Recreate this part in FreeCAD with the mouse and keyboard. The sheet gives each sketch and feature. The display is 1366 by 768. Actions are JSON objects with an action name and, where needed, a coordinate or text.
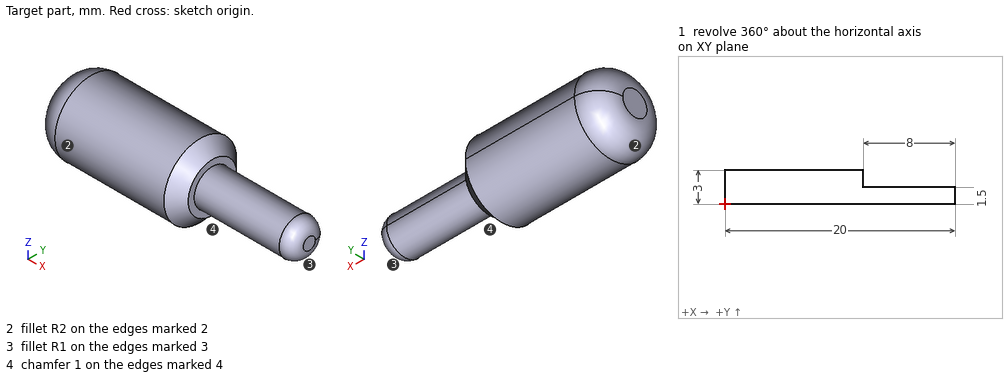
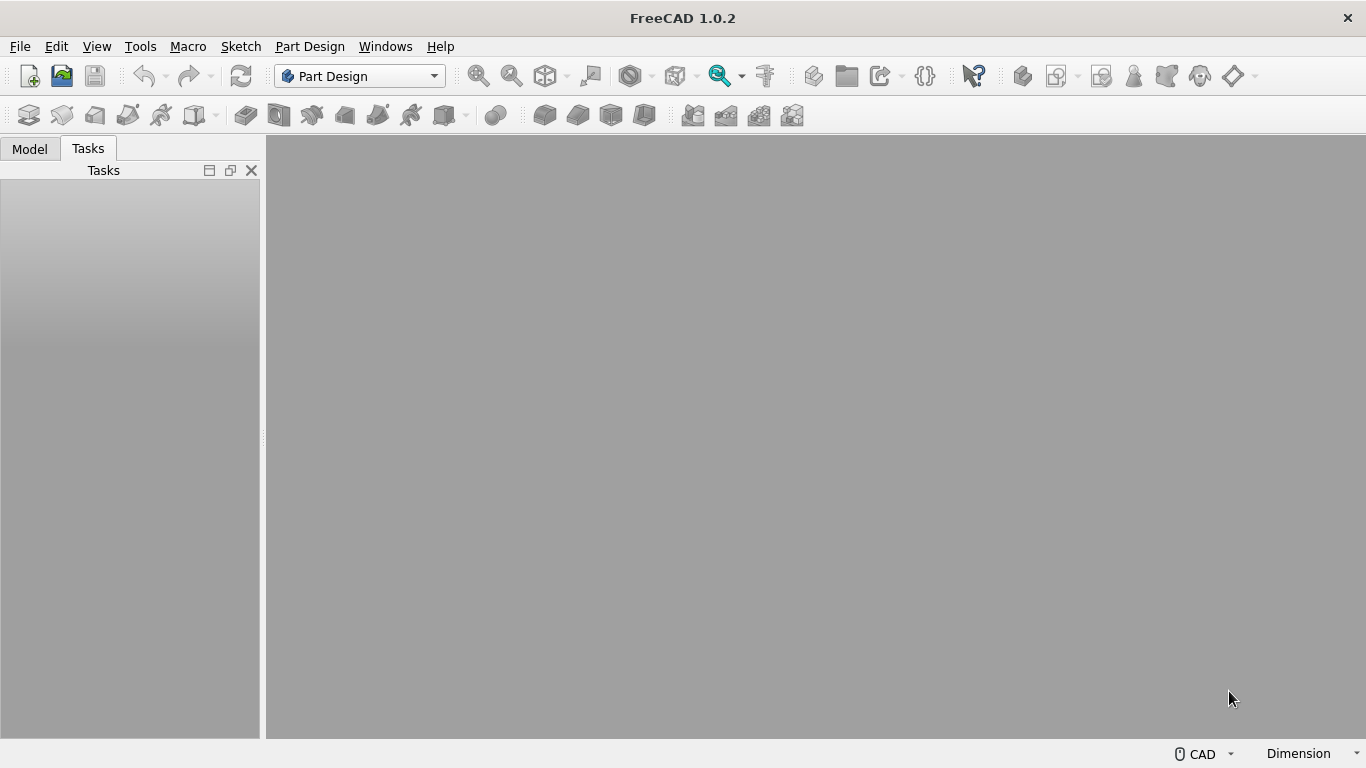
{"action": "key", "text": "ctrl+n"}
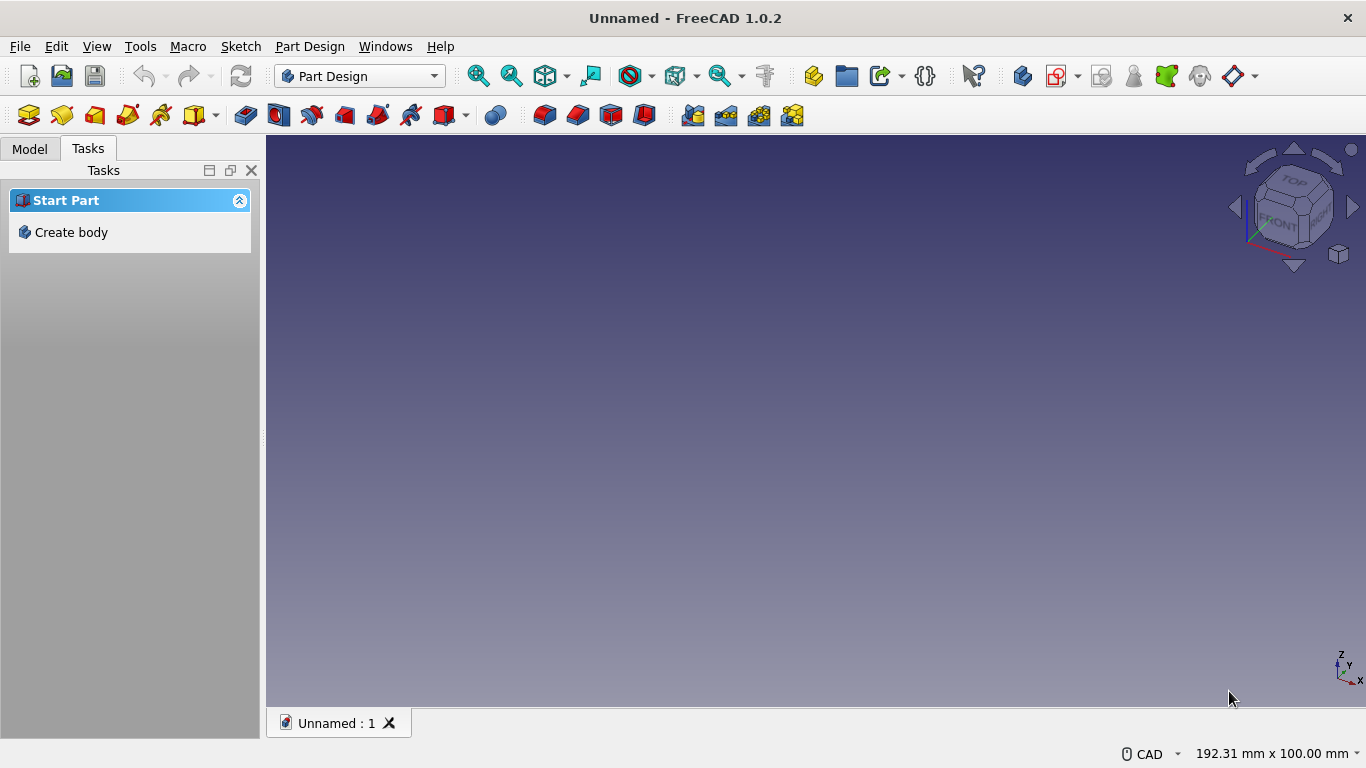
{"action": "left_click", "coordinate": [1056, 76]}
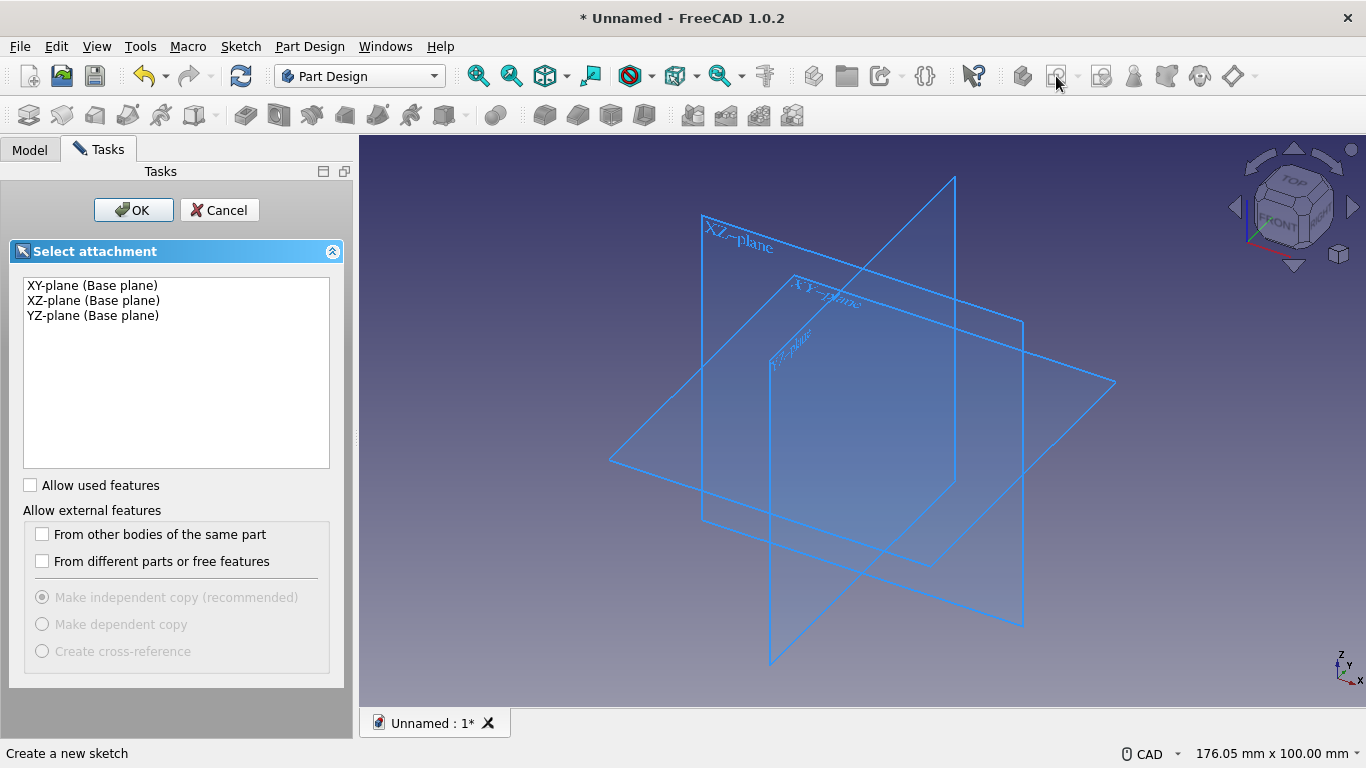
{"action": "left_click", "coordinate": [84, 286]}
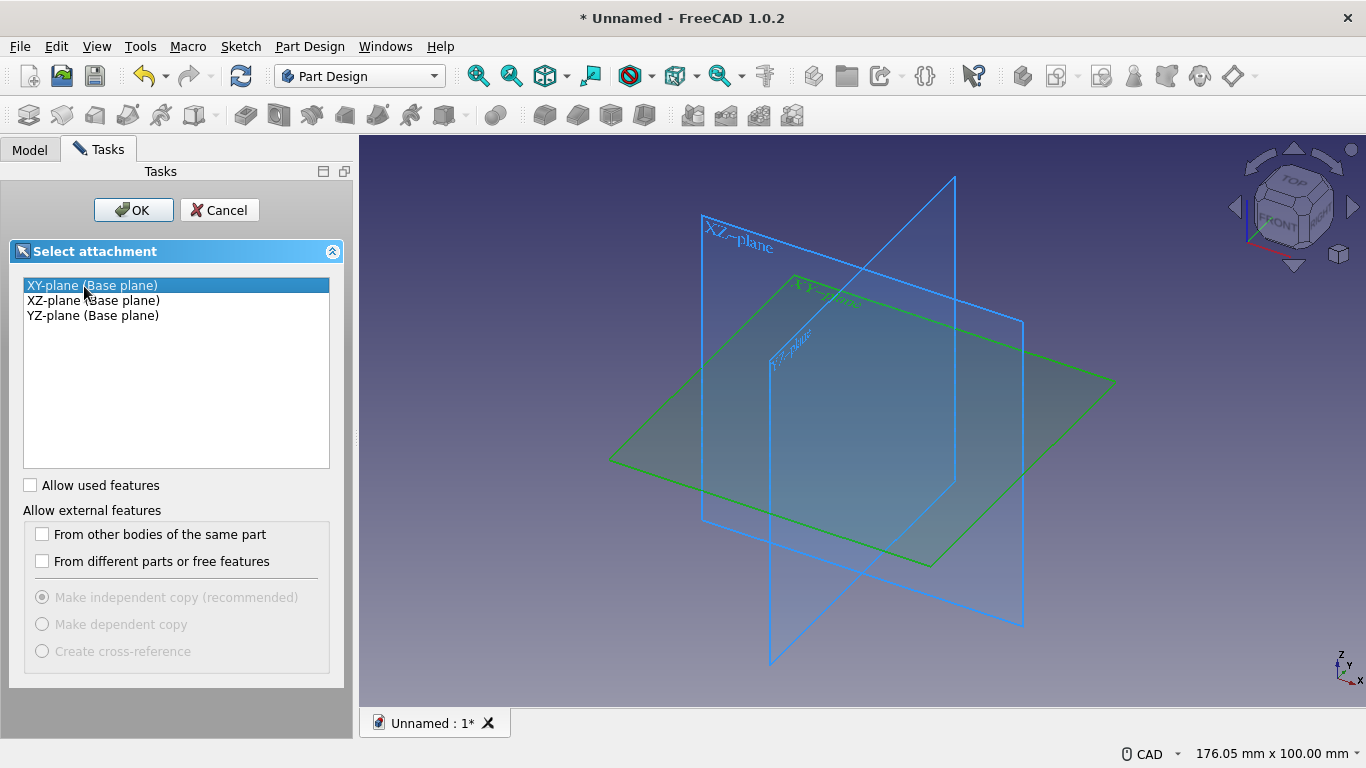
{"action": "left_click", "coordinate": [134, 210]}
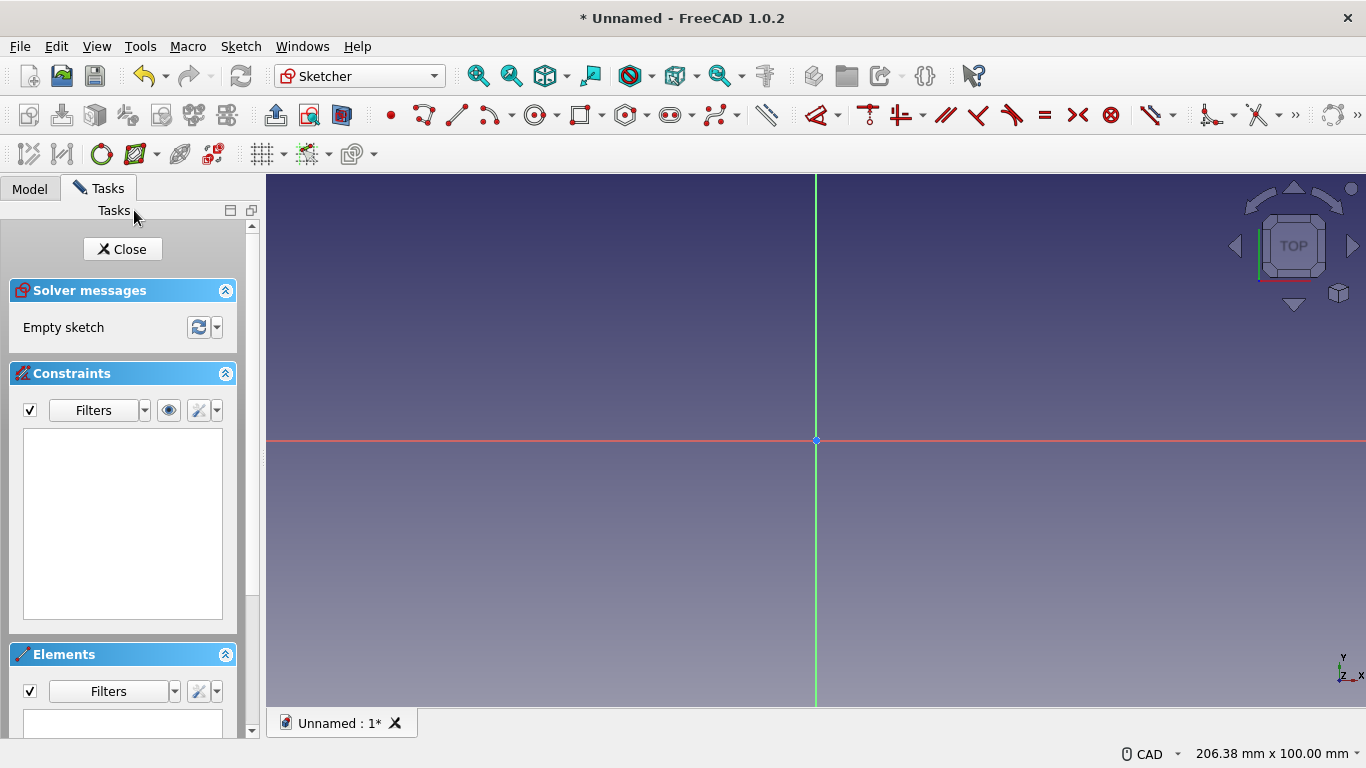
{"action": "scroll", "coordinate": [893, 431], "scroll_direction": "up", "scroll_amount": 9}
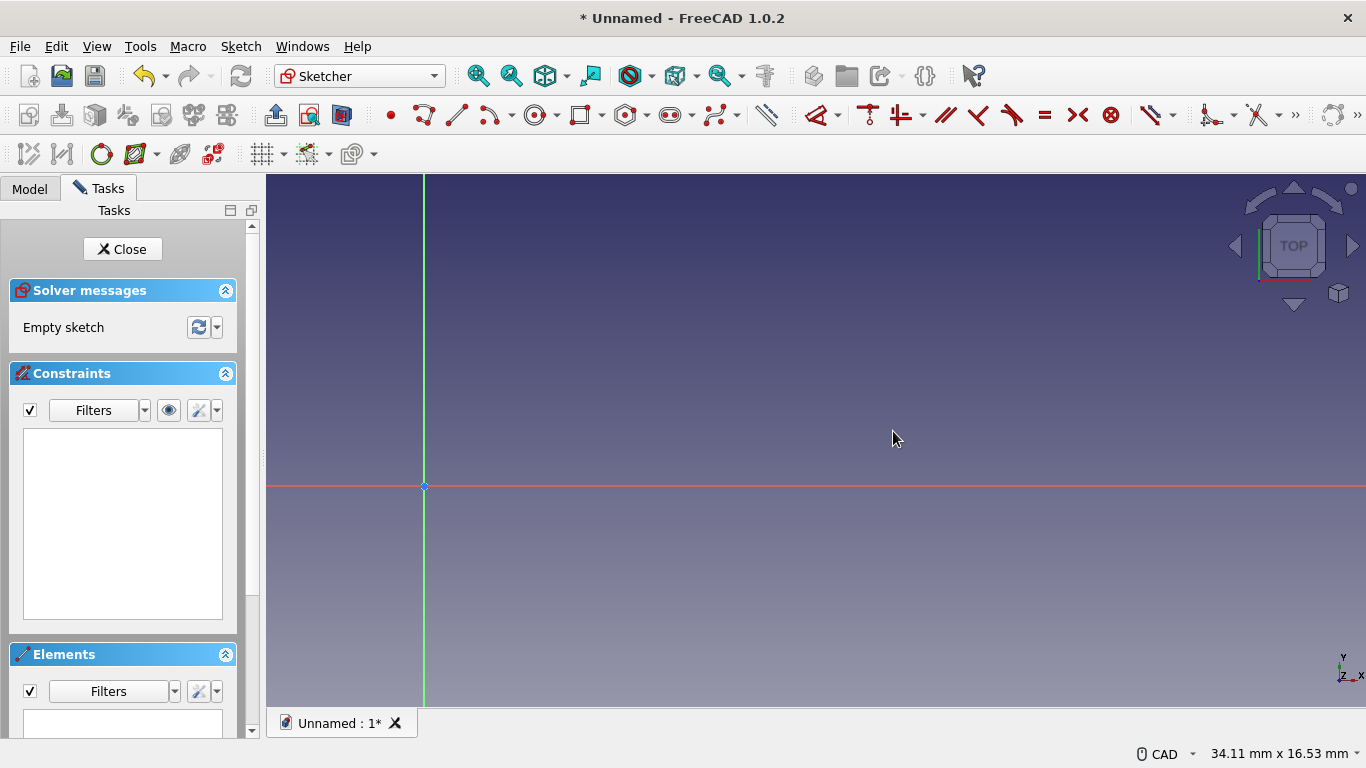
{"action": "key", "text": "g m"}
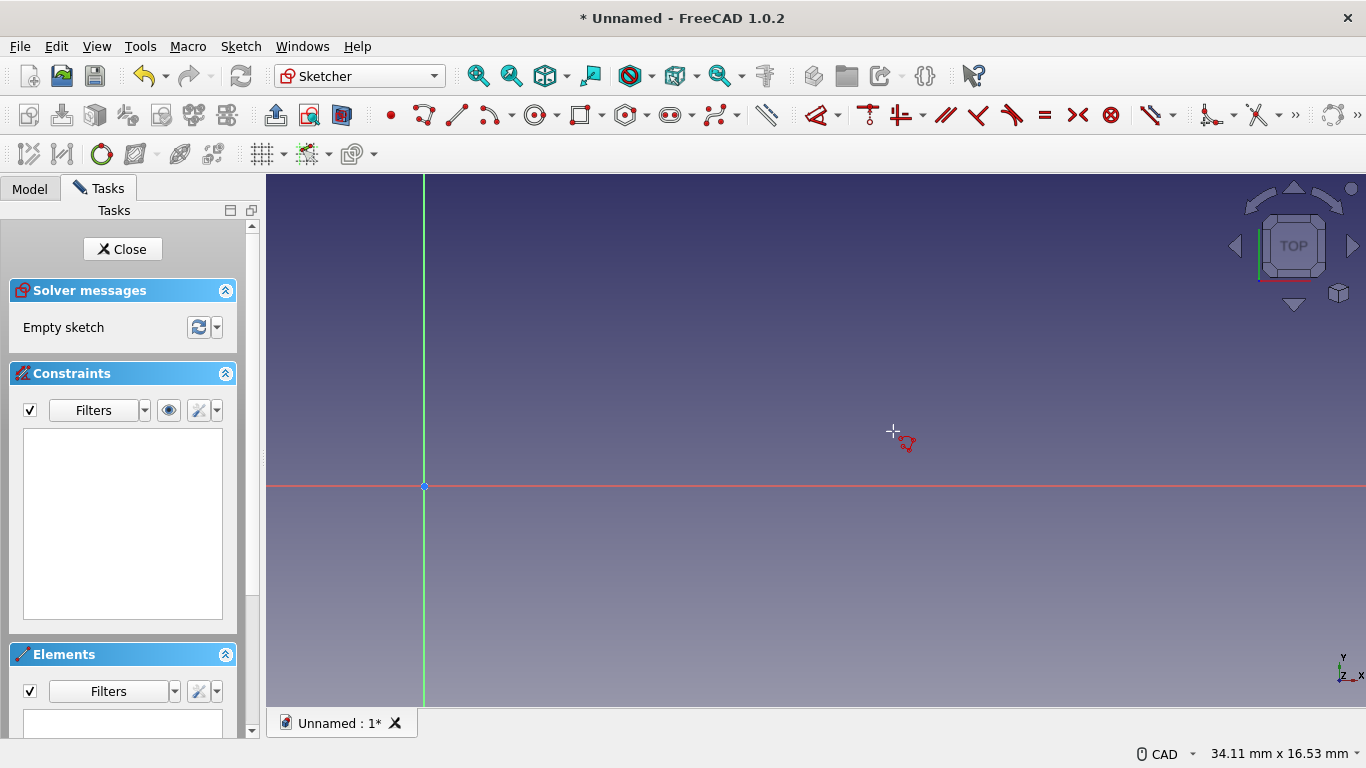
{"action": "left_click", "coordinate": [424, 486]}
{"action": "left_click", "coordinate": [1069, 477]}
{"action": "left_click", "coordinate": [1069, 438]}
{"action": "left_click", "coordinate": [811, 438]}
{"action": "left_click", "coordinate": [811, 389]}
{"action": "left_click", "coordinate": [433, 389]}
{"action": "left_click", "coordinate": [424, 486]}
{"action": "key", "text": "Escape"}
{"action": "key", "text": "Escape"}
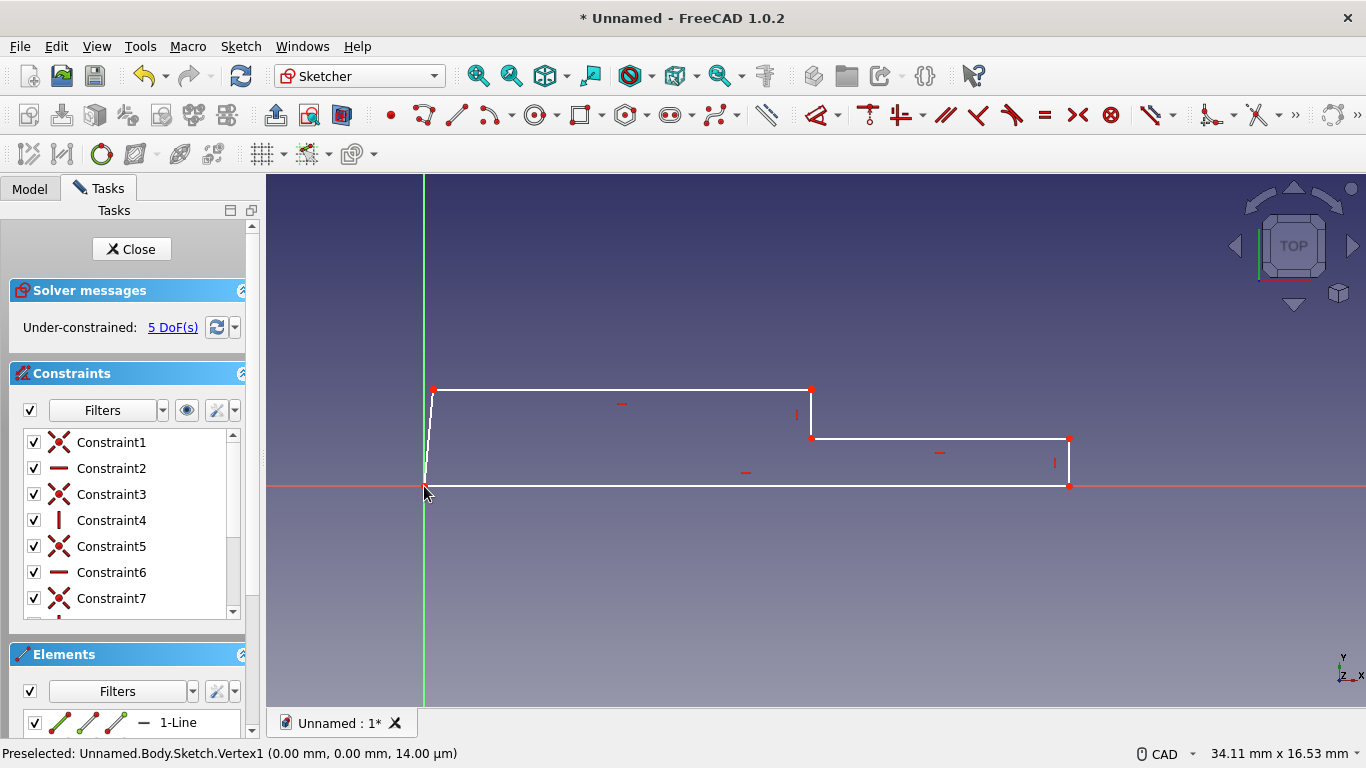
{"action": "left_click", "coordinate": [427, 457]}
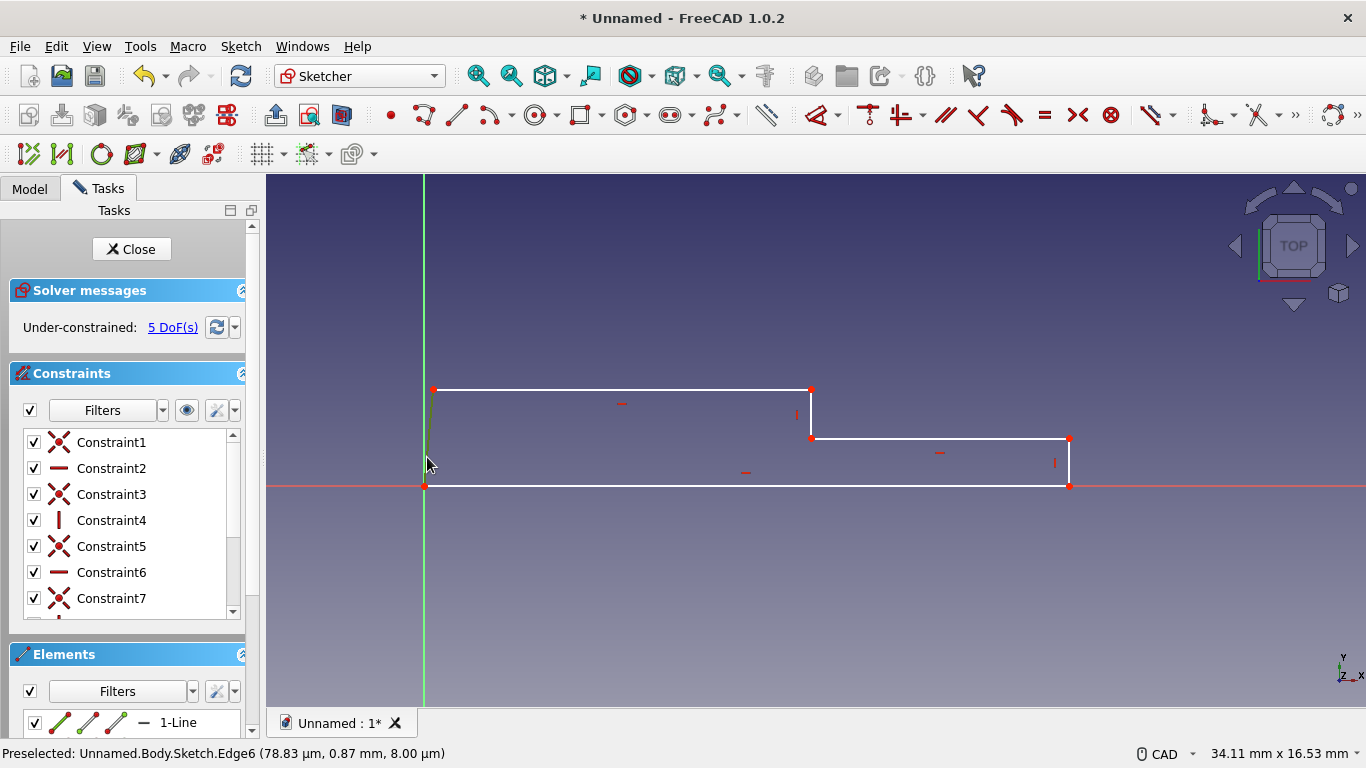
{"action": "key", "text": "v"}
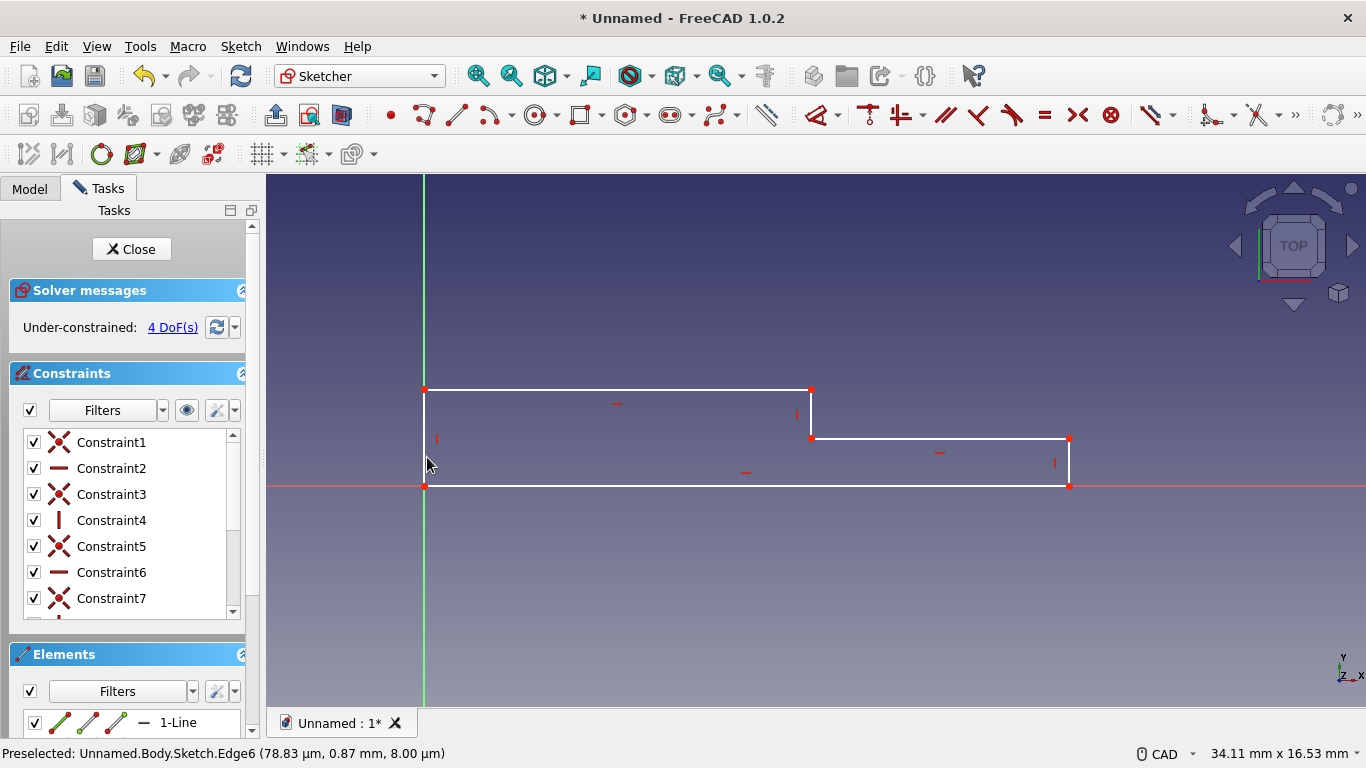
{"action": "left_click", "coordinate": [816, 116]}